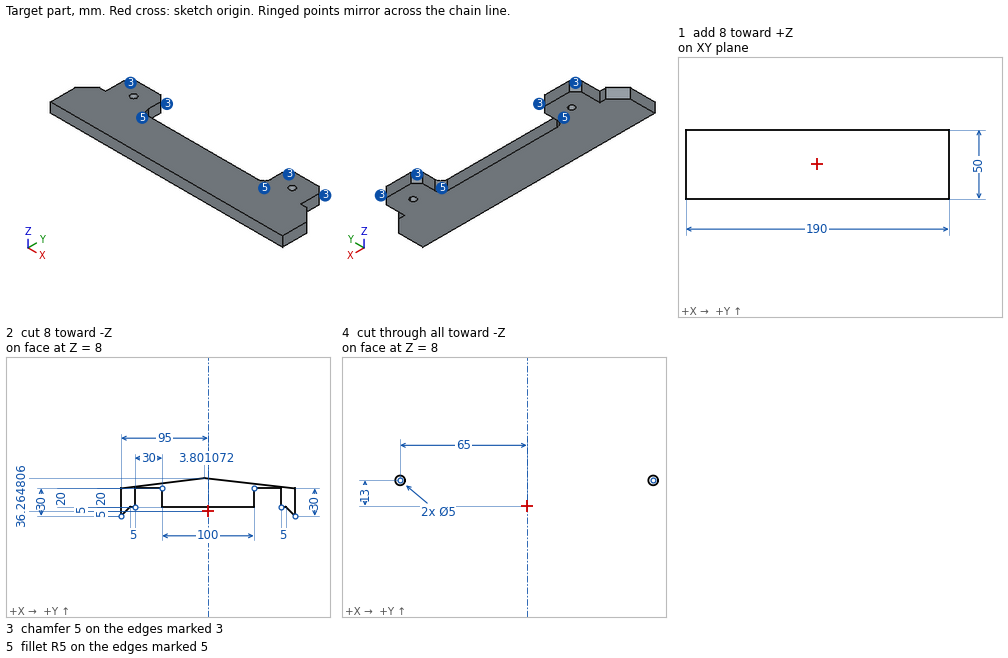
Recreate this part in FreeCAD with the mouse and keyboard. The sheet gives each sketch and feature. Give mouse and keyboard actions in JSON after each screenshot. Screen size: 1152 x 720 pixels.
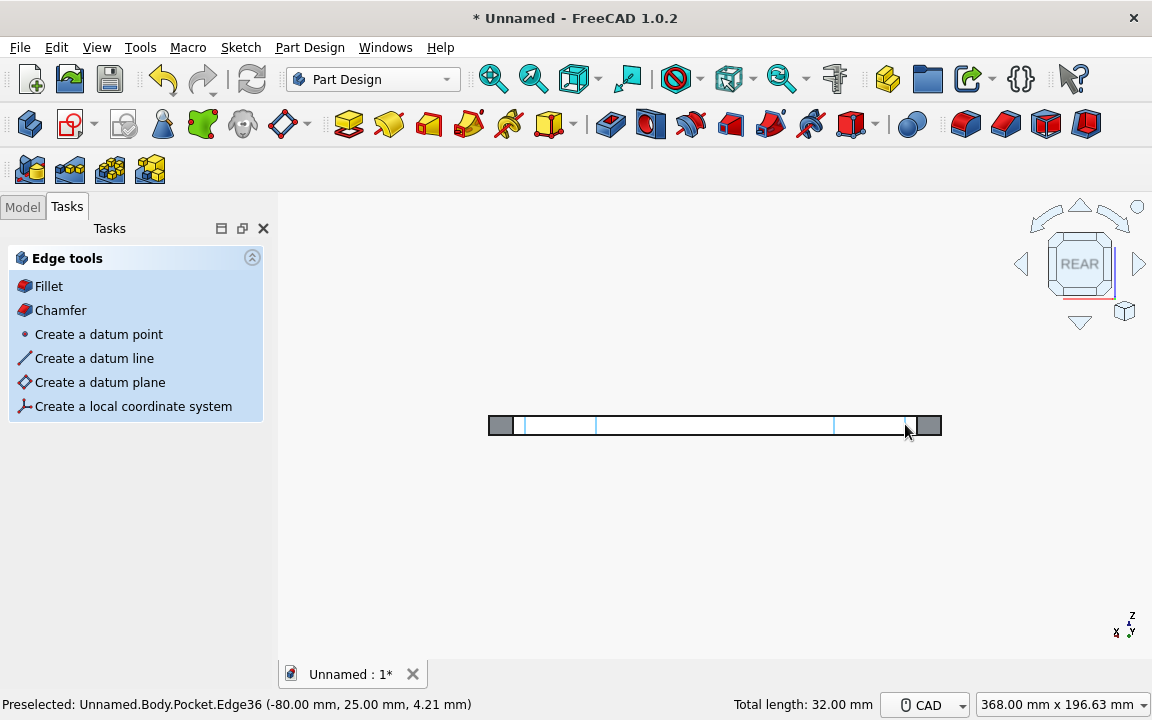
{"action": "left_click", "coordinate": [1006, 124]}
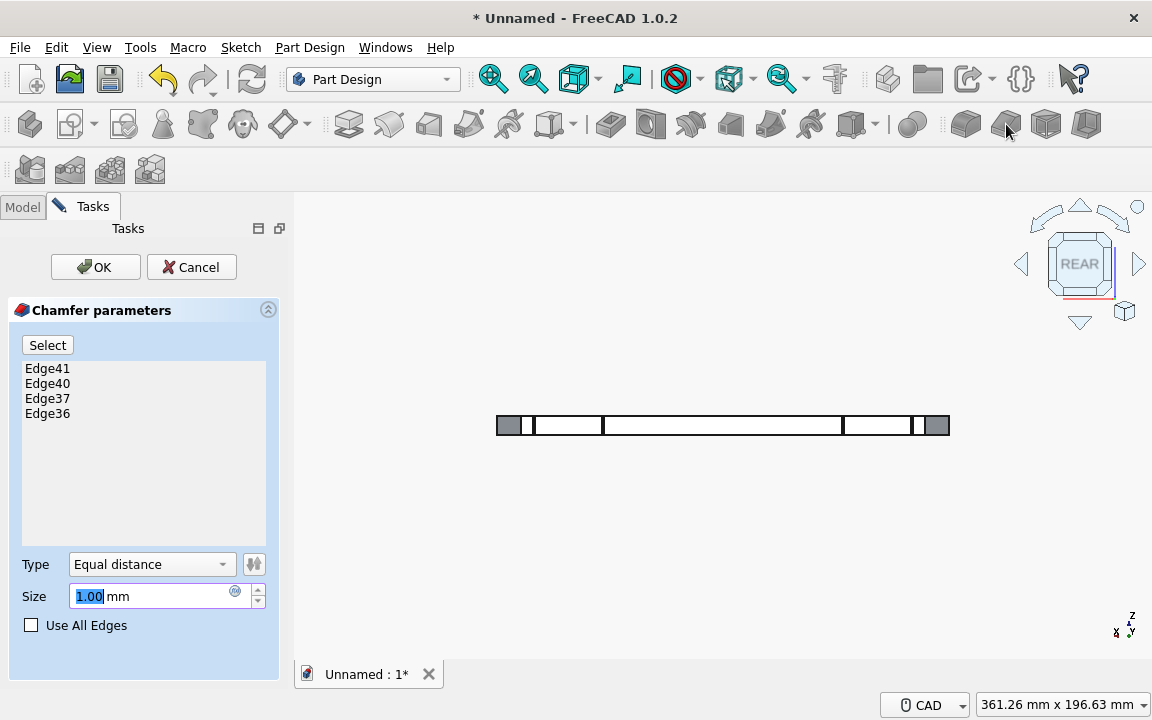
{"action": "type", "text": "5"}
{"action": "key", "text": "Tab"}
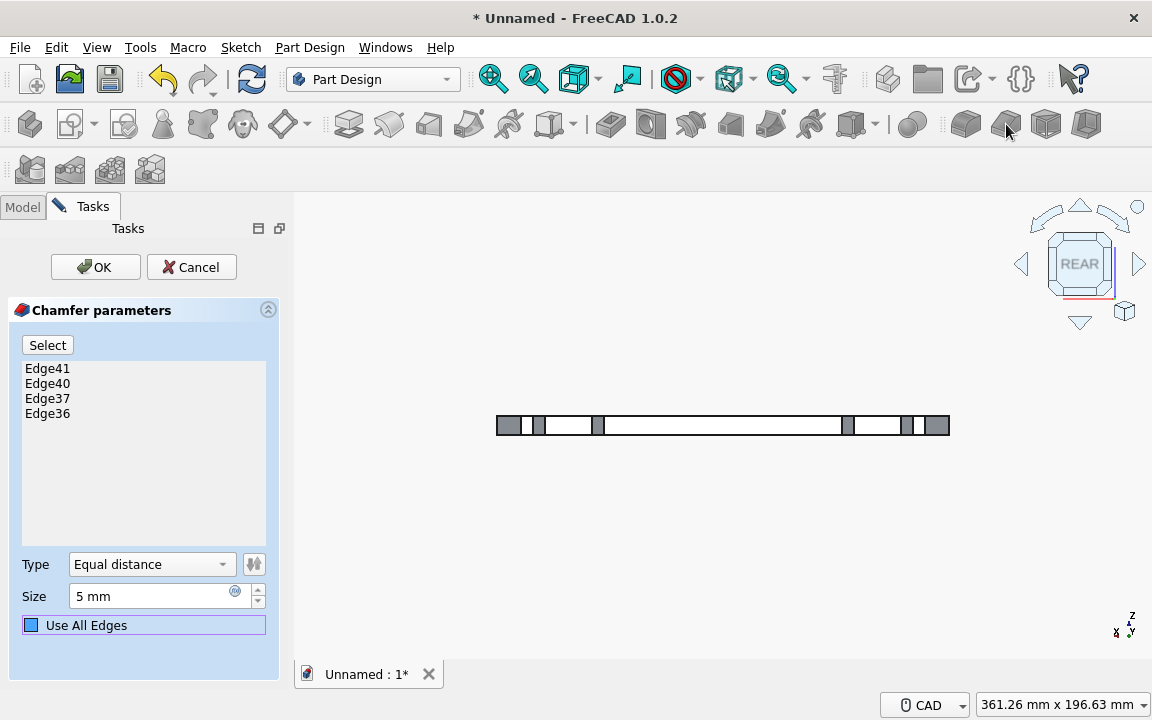
{"action": "left_click", "coordinate": [96, 267]}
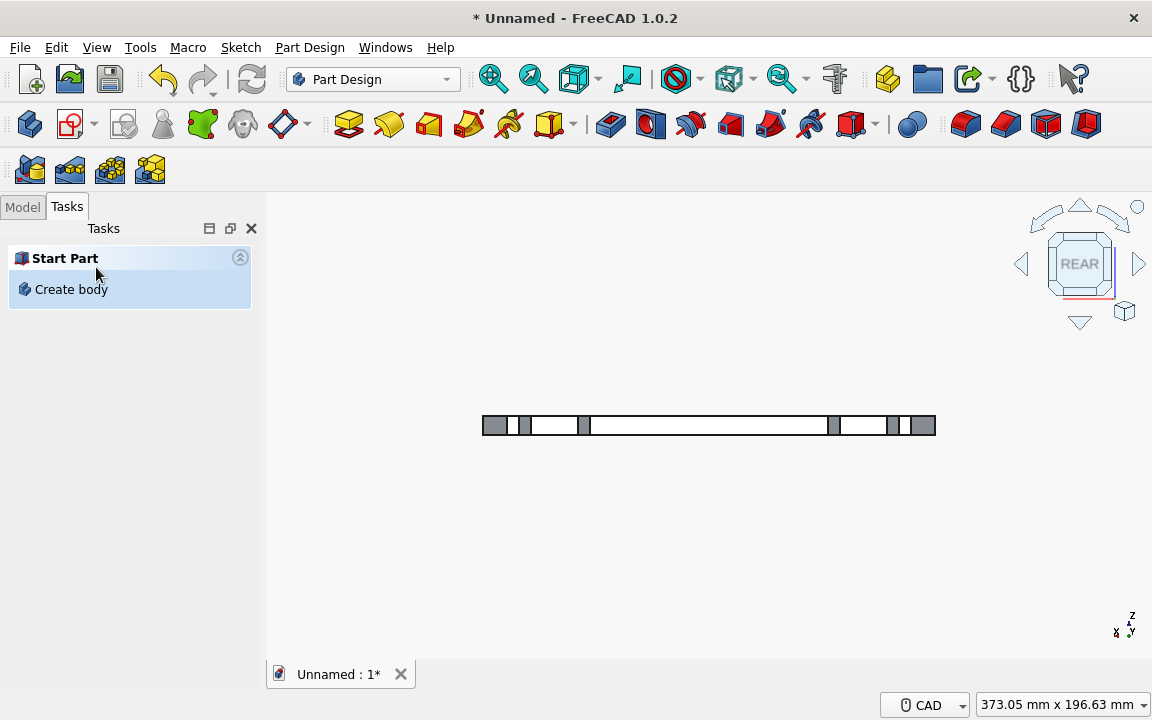
{"action": "key", "text": "0"}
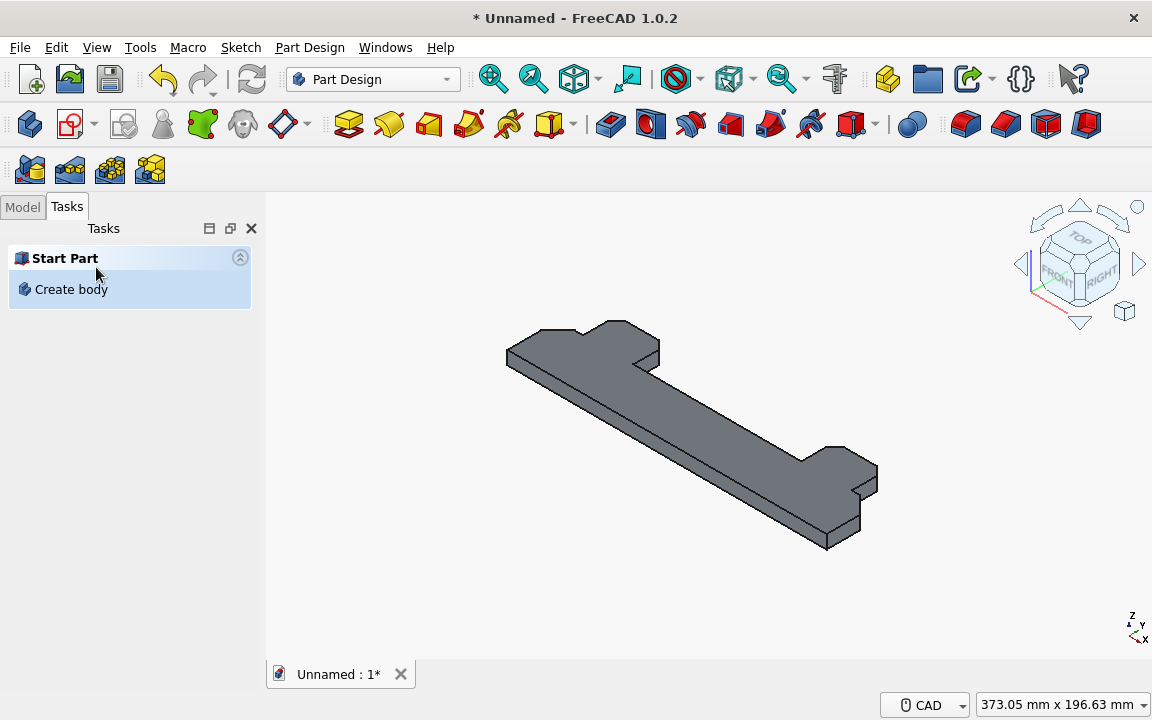
{"action": "left_click", "coordinate": [606, 371]}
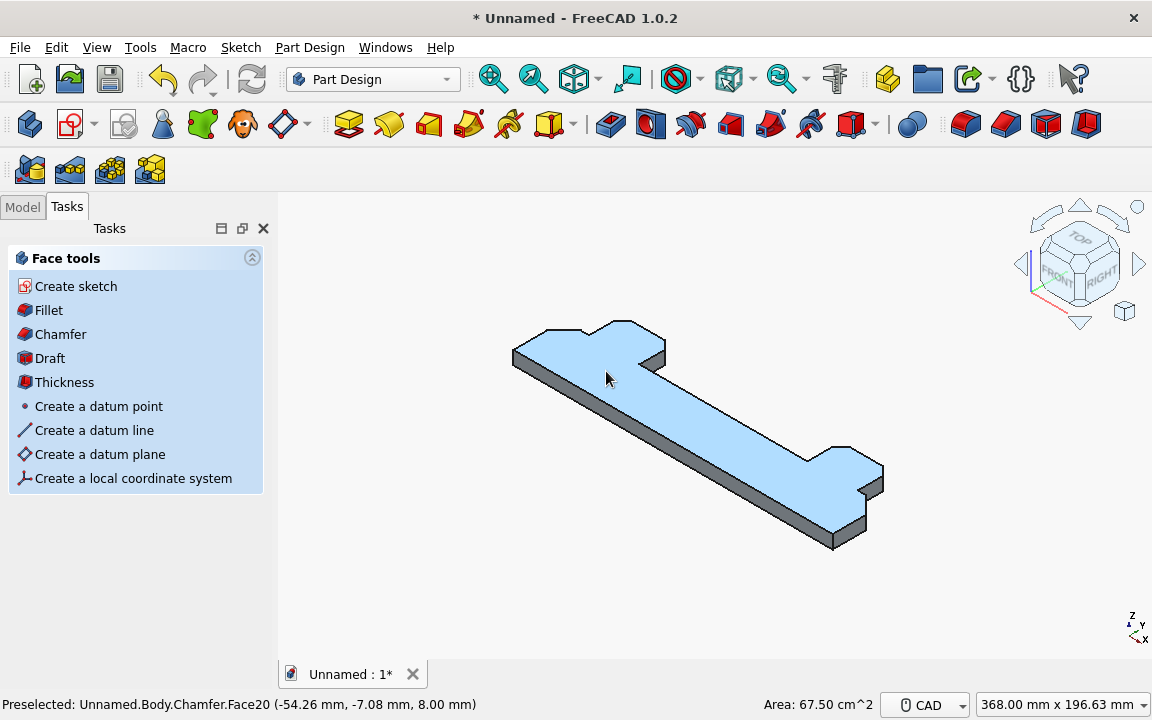
{"action": "left_click", "coordinate": [70, 124]}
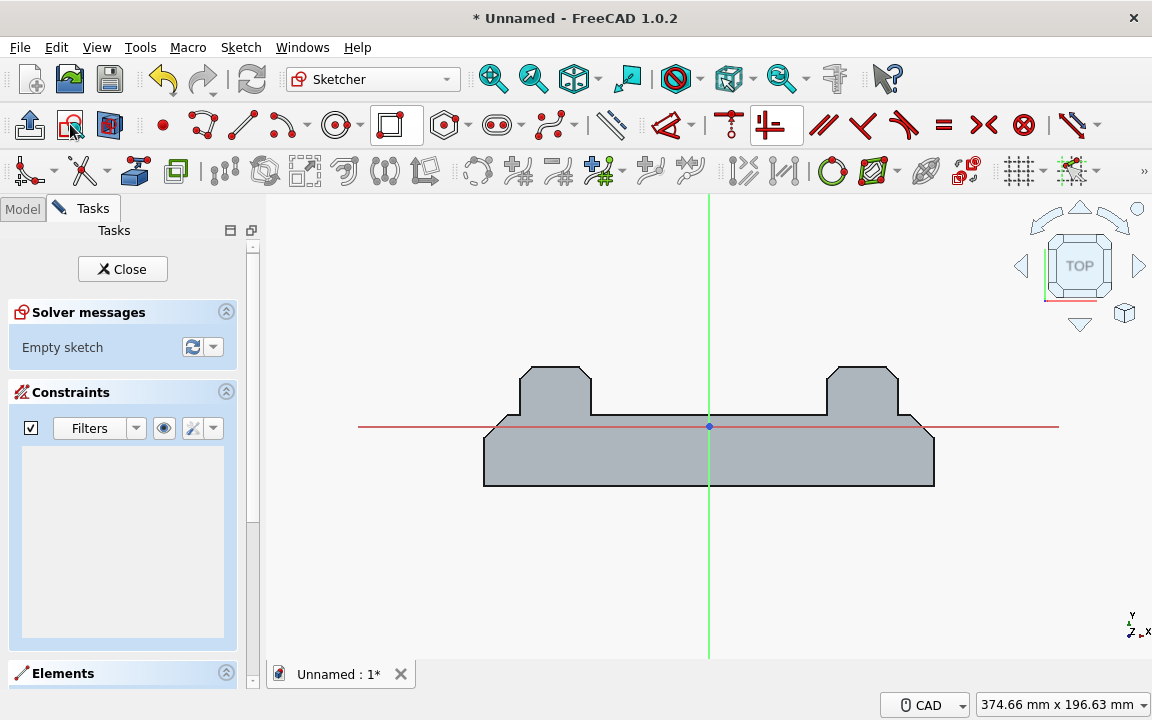
{"action": "scroll", "coordinate": [848, 371], "scroll_direction": "up", "scroll_amount": 2}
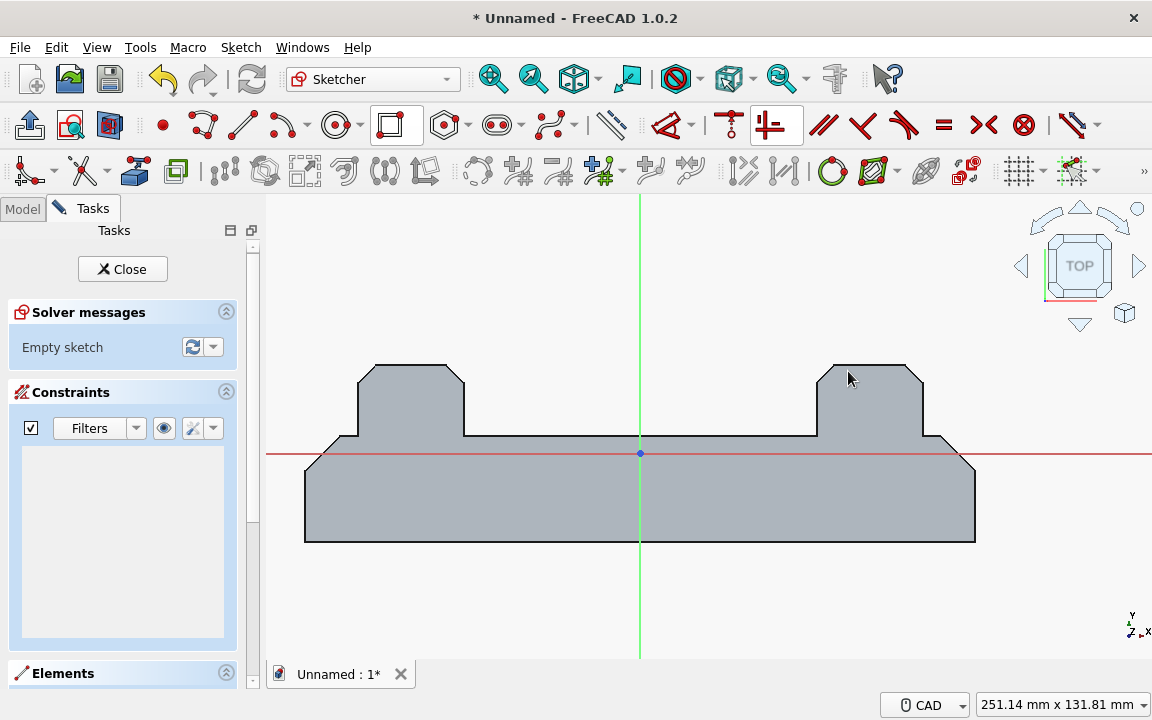
{"action": "left_click", "coordinate": [336, 126]}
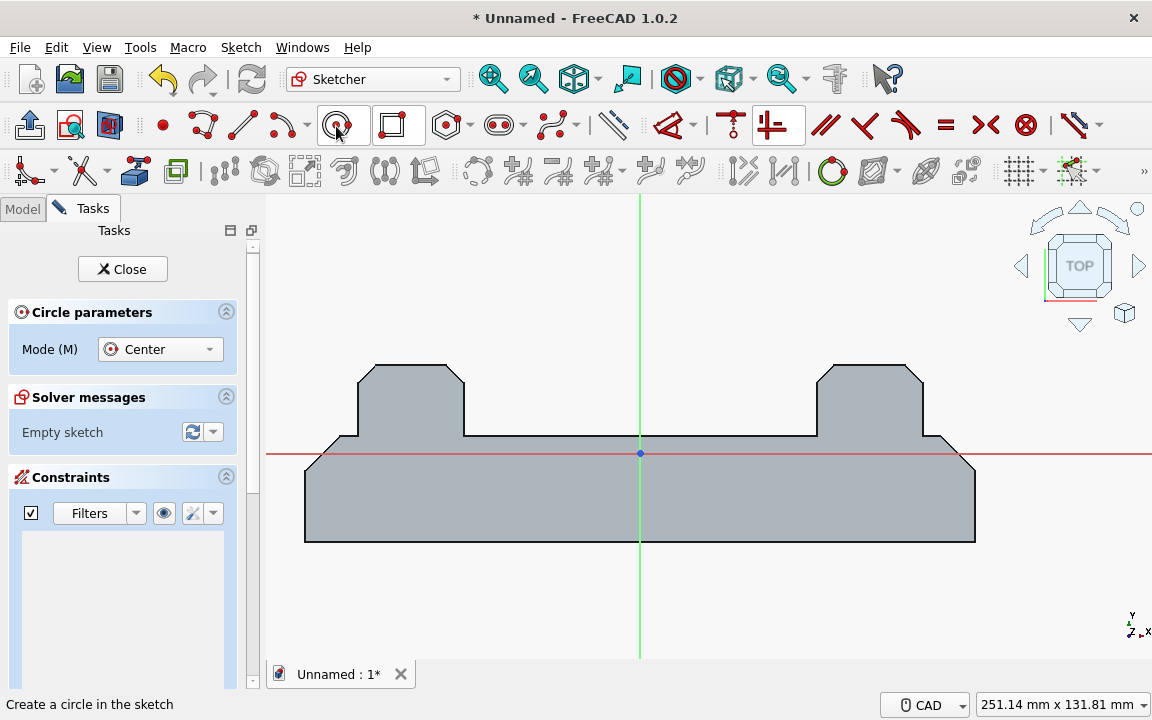
{"action": "scroll", "coordinate": [411, 408], "scroll_direction": "up", "scroll_amount": 5}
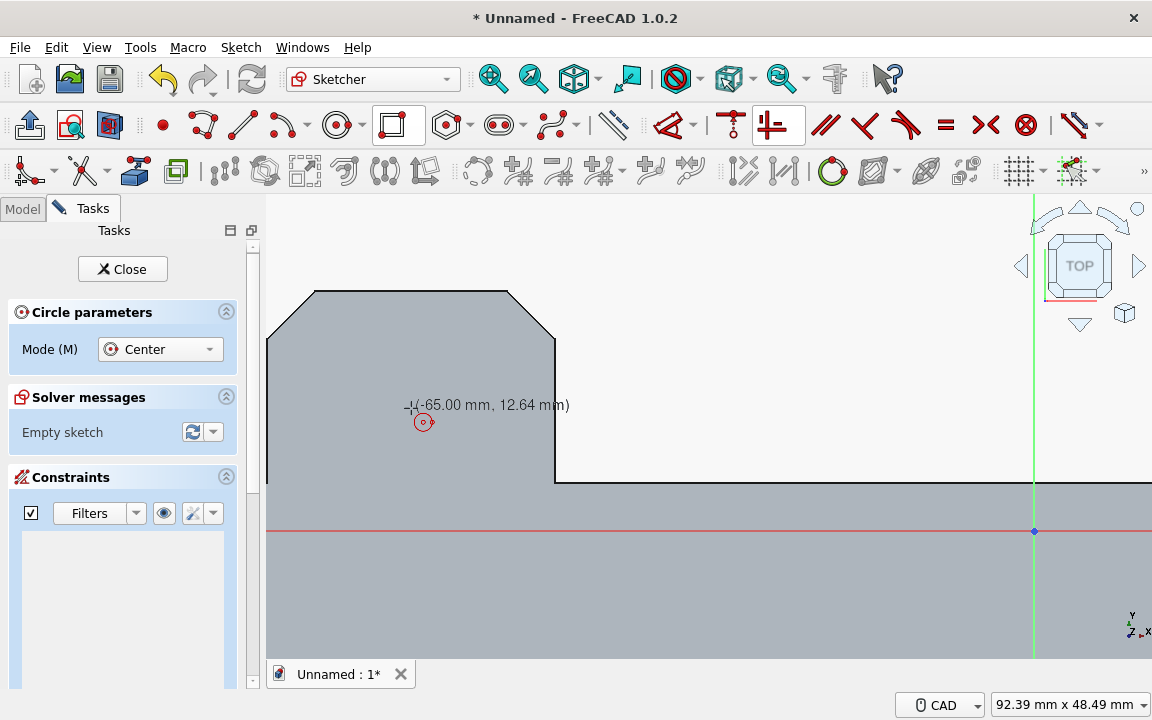
{"action": "left_click", "coordinate": [411, 407]}
{"action": "mouse_move", "coordinate": [428, 390]}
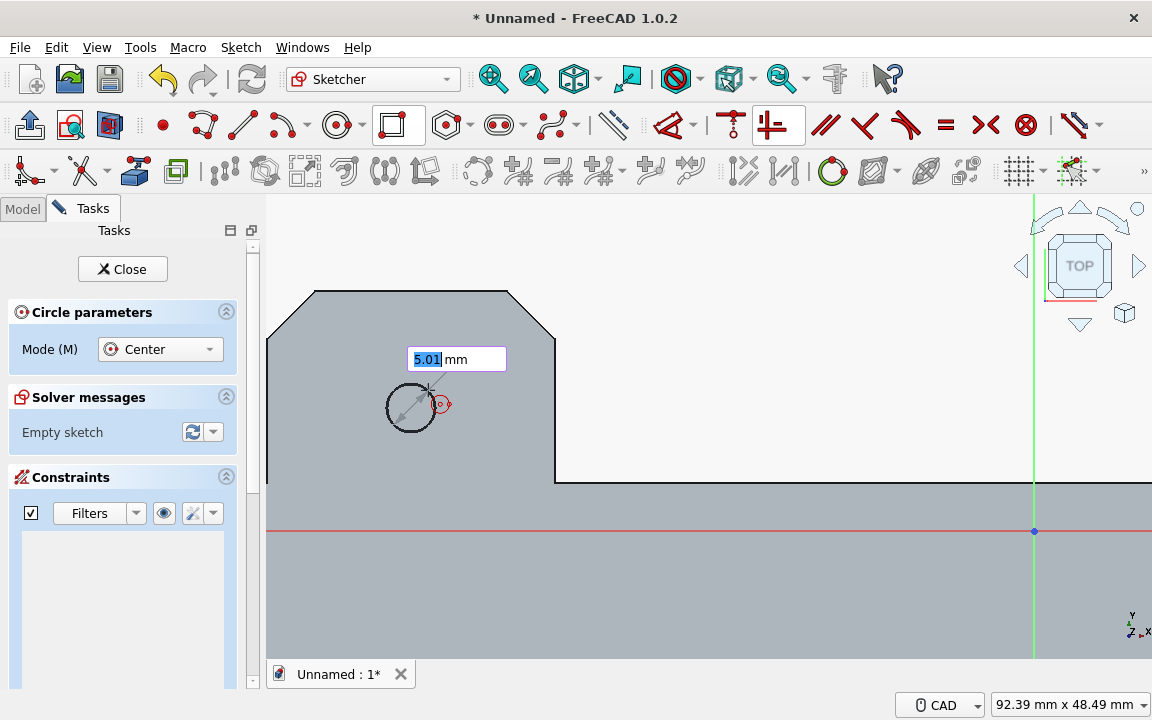
{"action": "type", "text": "5"}
{"action": "key", "text": "Return"}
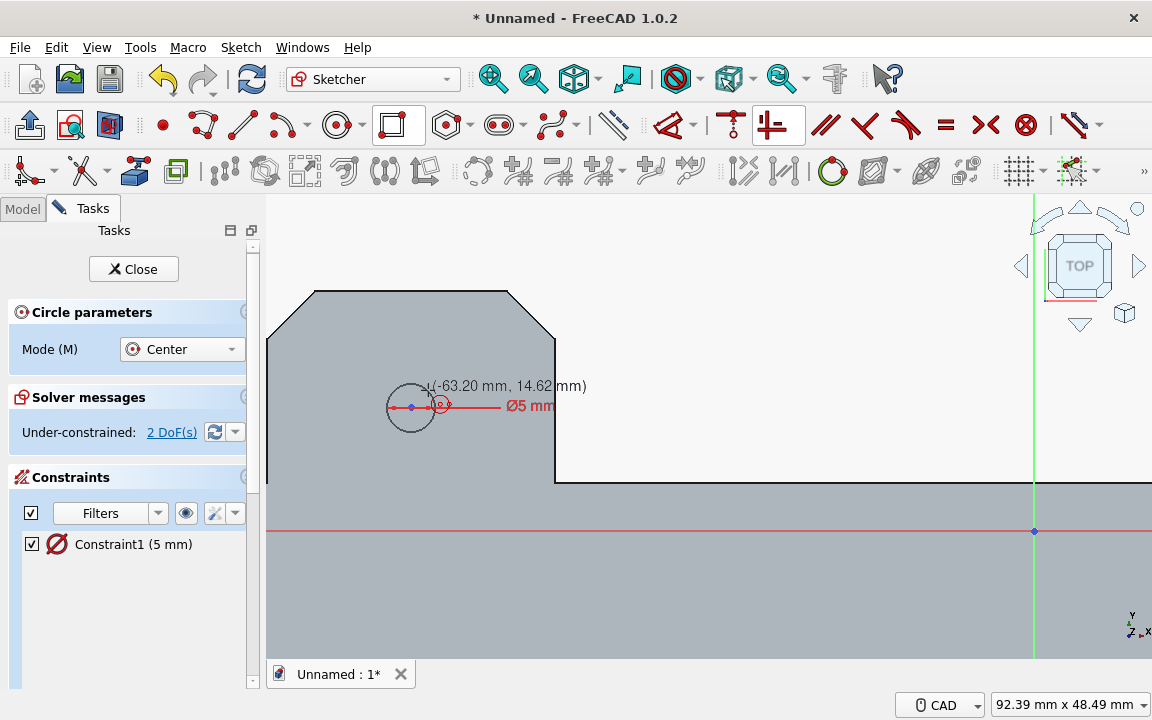
{"action": "scroll", "coordinate": [411, 409], "scroll_direction": "down", "scroll_amount": 5}